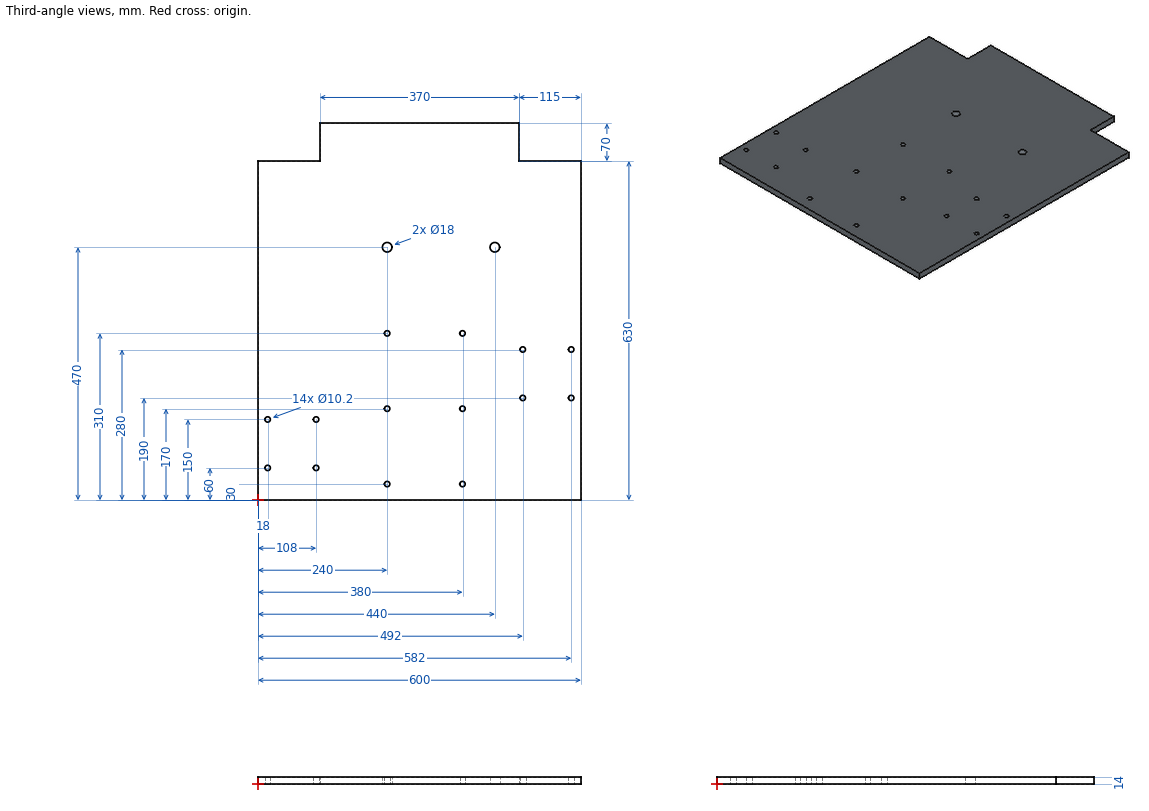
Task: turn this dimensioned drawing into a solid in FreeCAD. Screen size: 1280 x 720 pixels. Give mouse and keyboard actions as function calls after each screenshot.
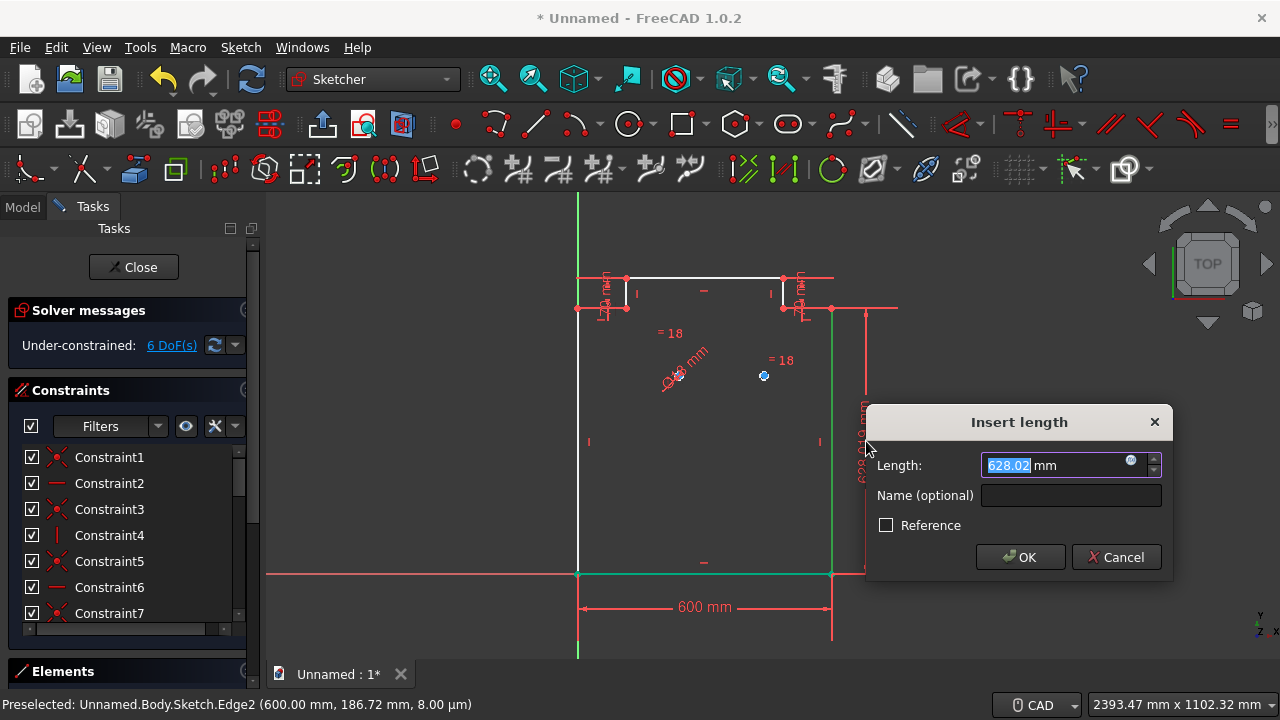
text(630)
key(Return)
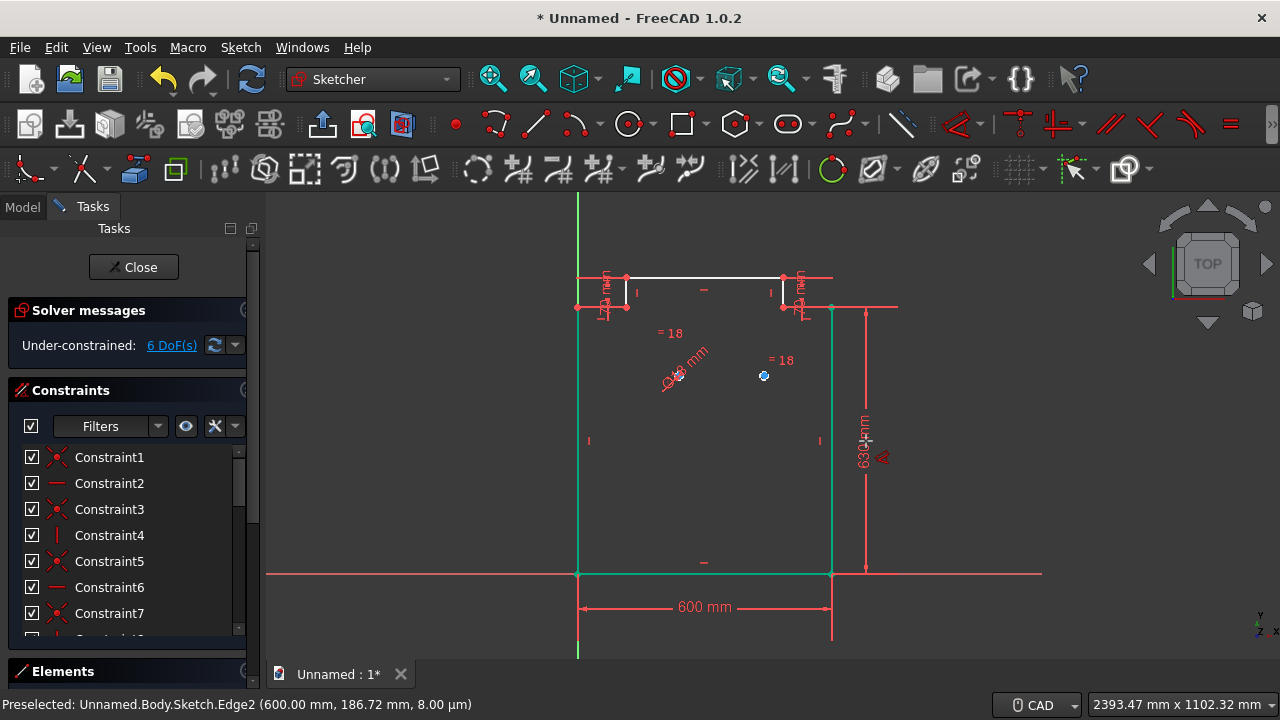
click(817, 307)
click(807, 341)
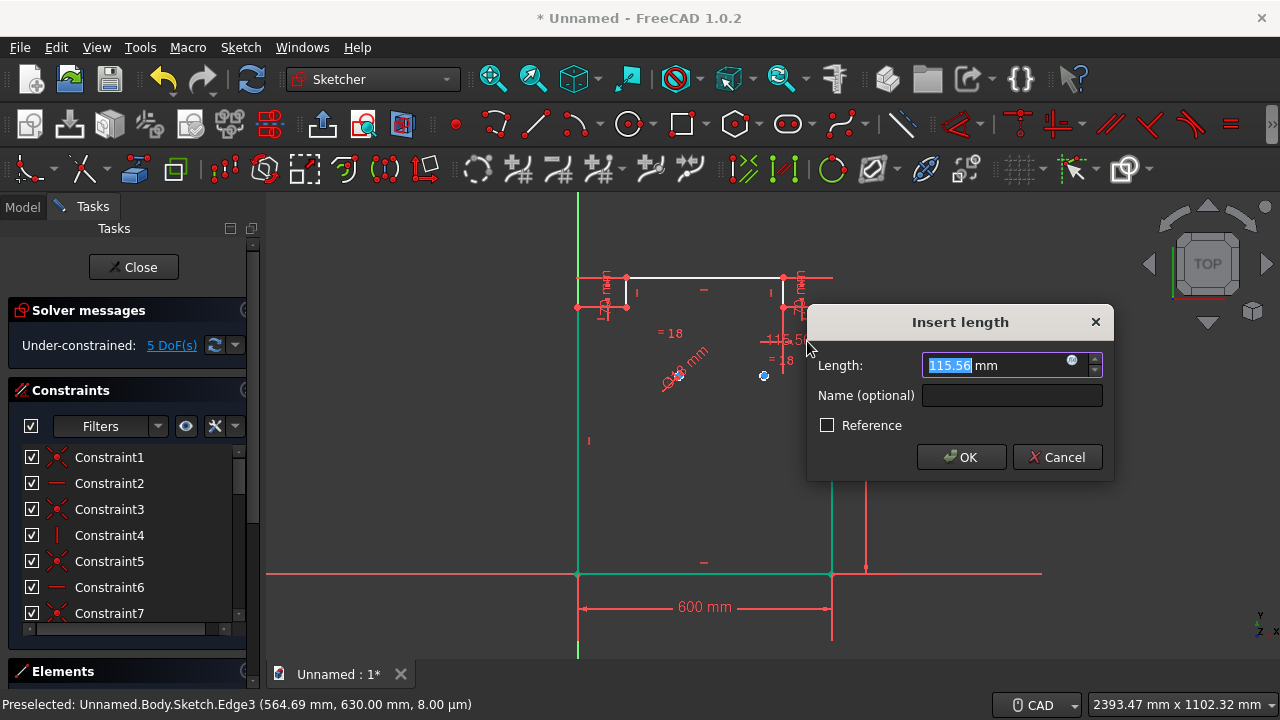
text(115)
key(Return)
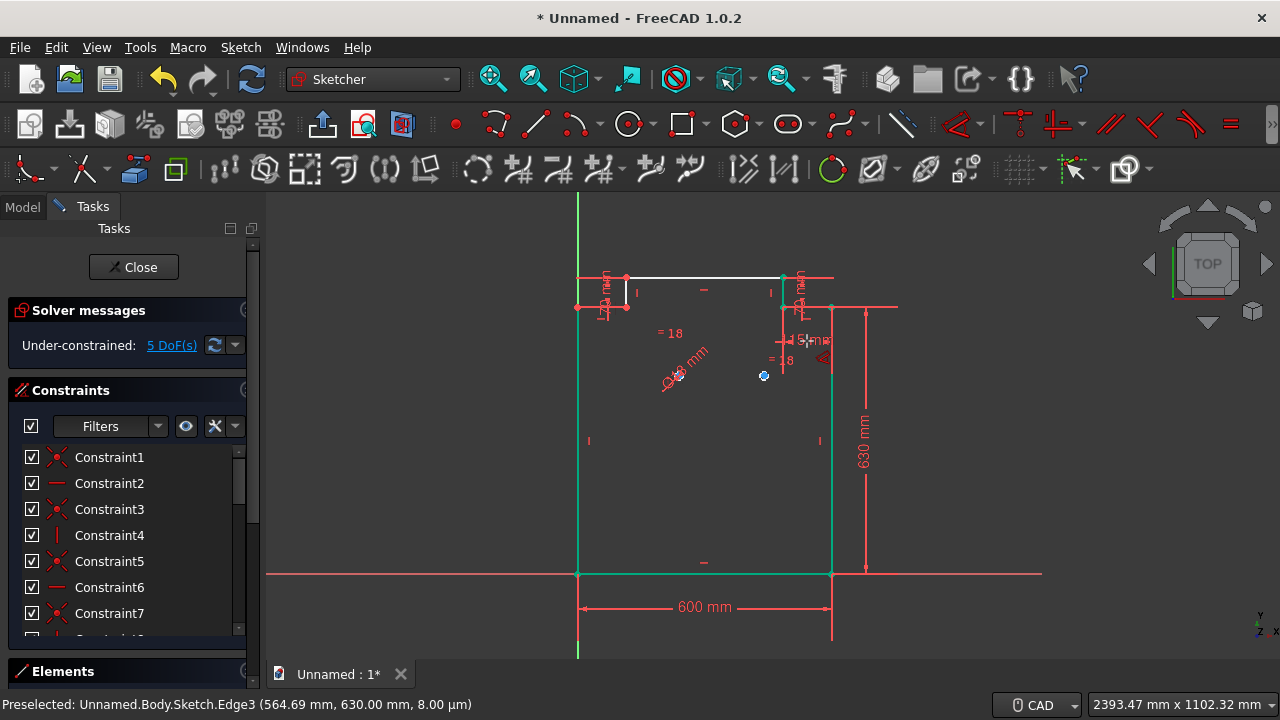
click(736, 278)
click(705, 244)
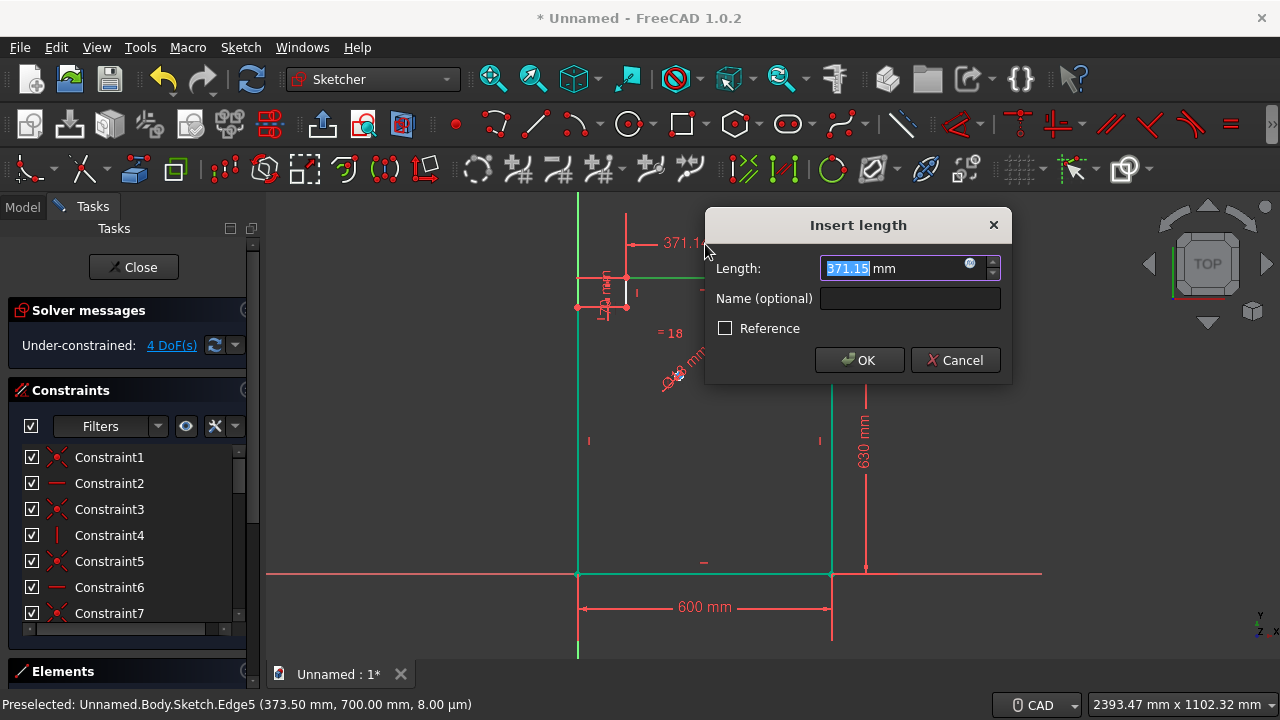
text(370)
key(Return)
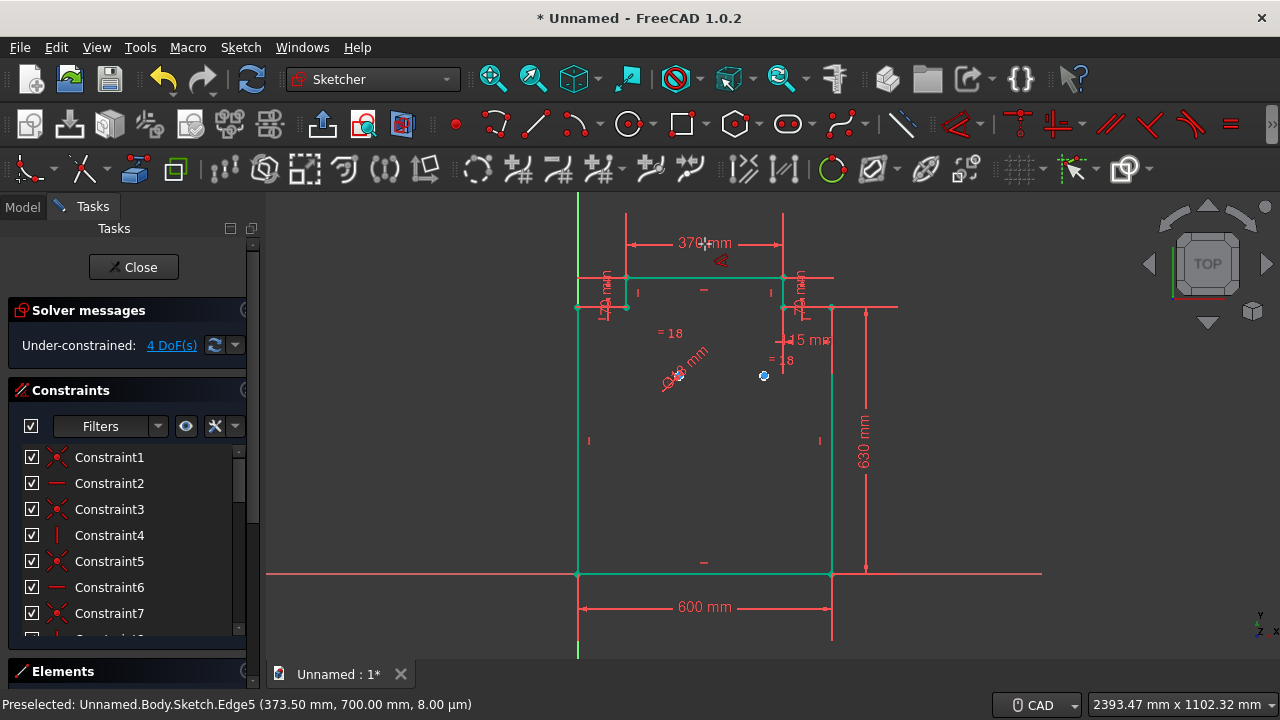
click(679, 376)
click(628, 608)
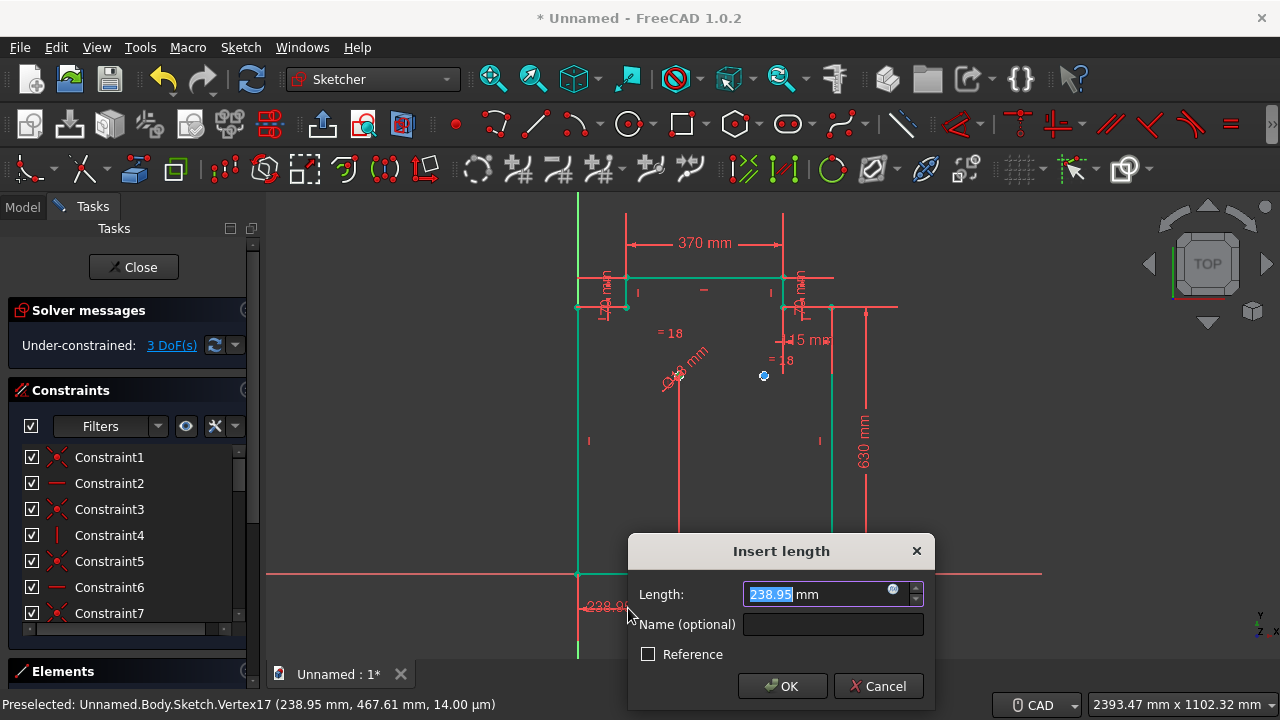
text(240)
key(Return)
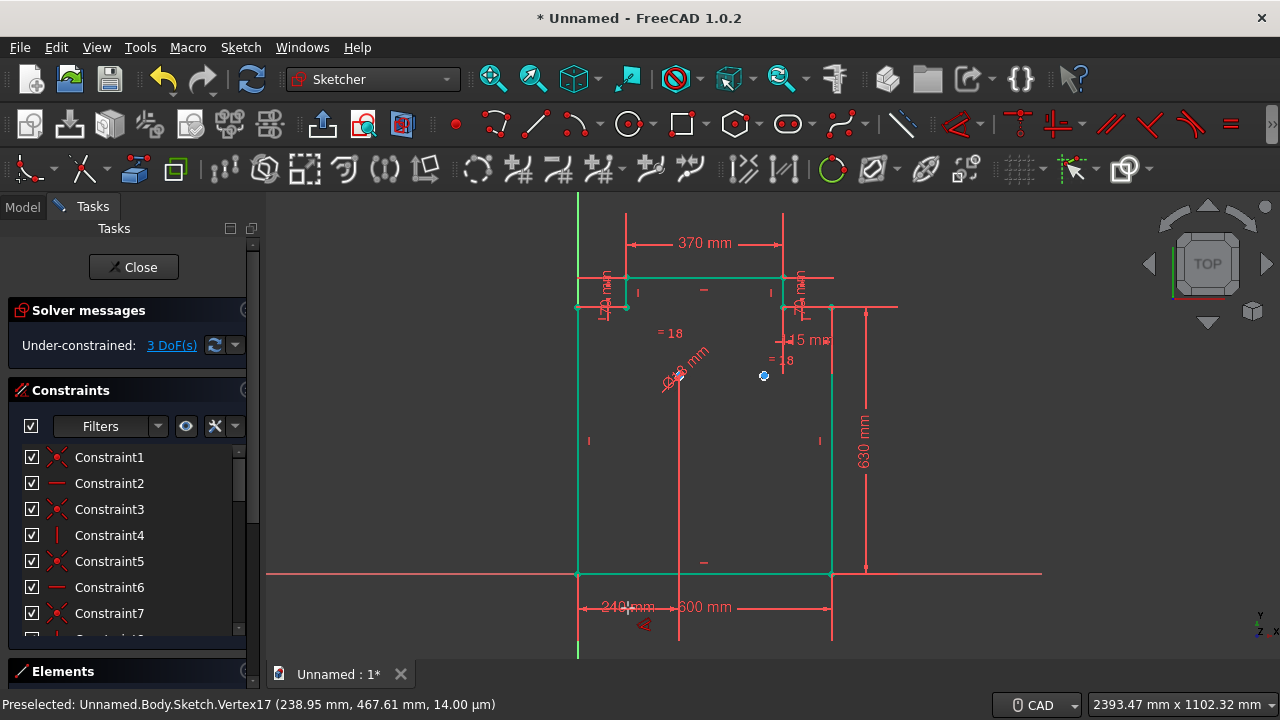
click(679, 376)
click(544, 475)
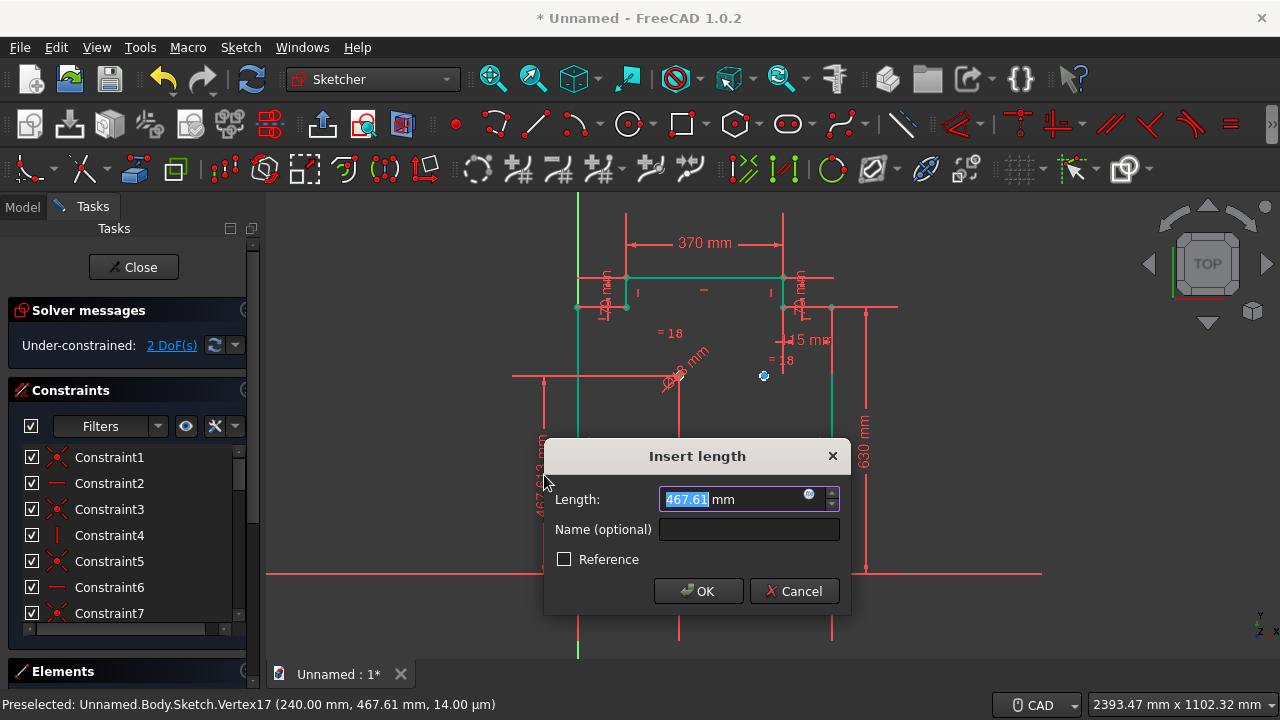
text(470)
key(Return)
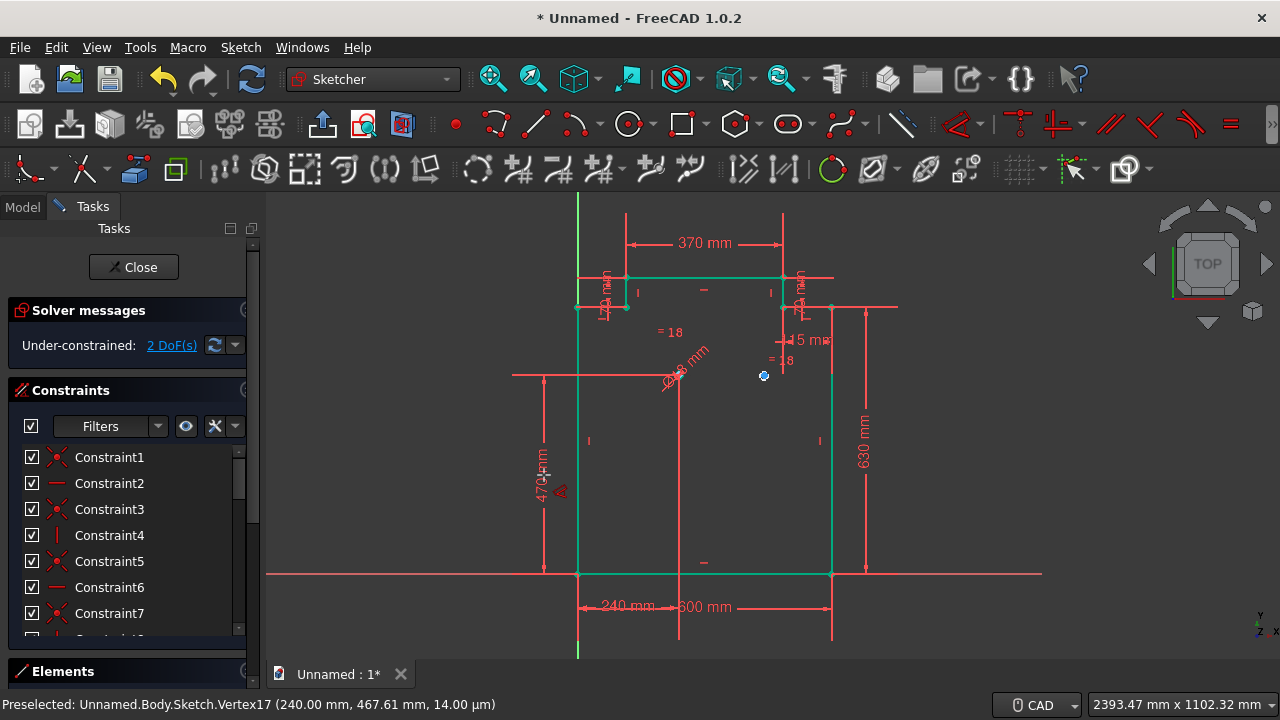
click(764, 376)
click(671, 342)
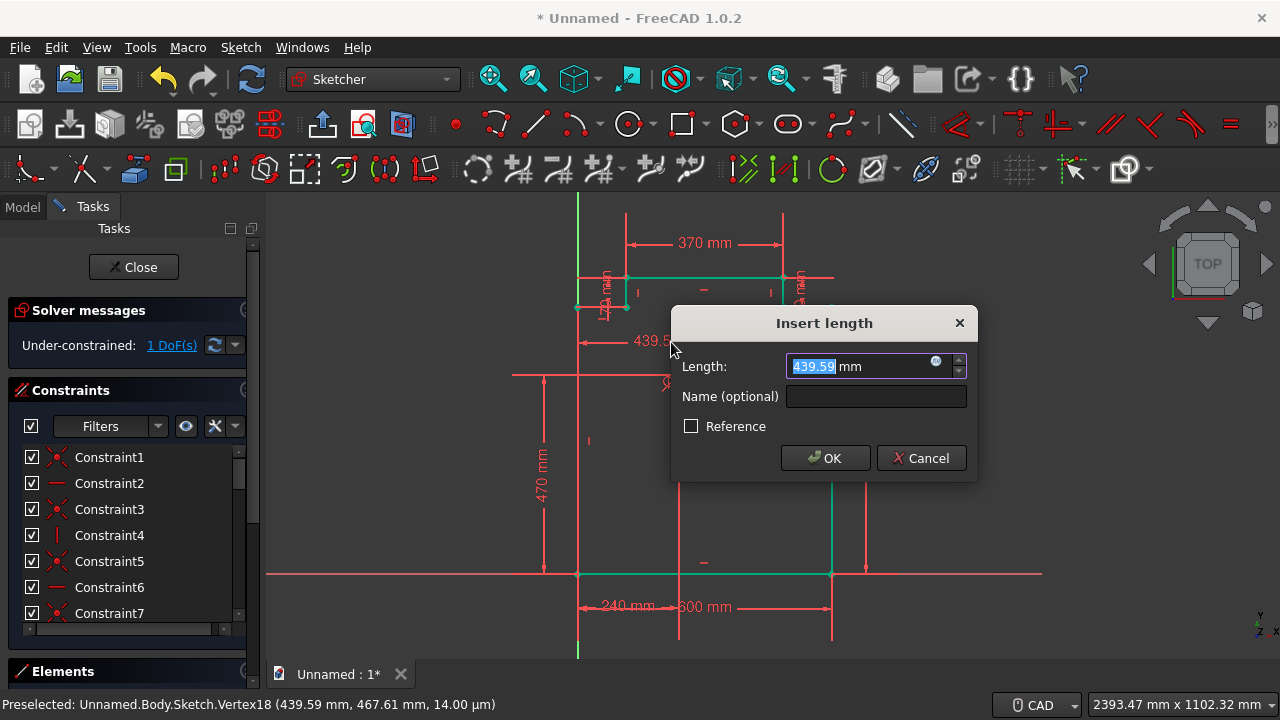
text(440)
key(Return)